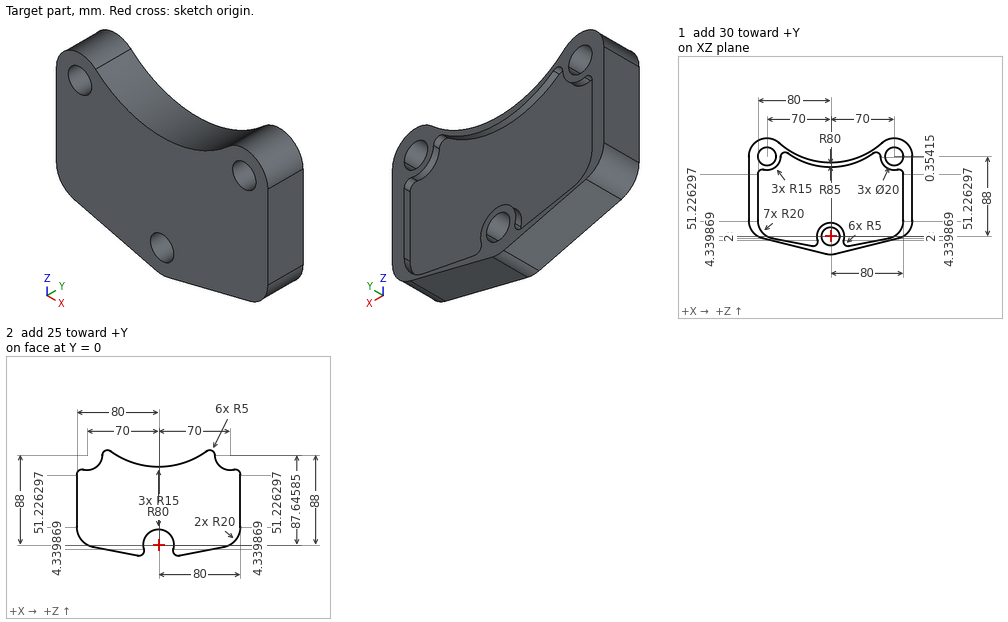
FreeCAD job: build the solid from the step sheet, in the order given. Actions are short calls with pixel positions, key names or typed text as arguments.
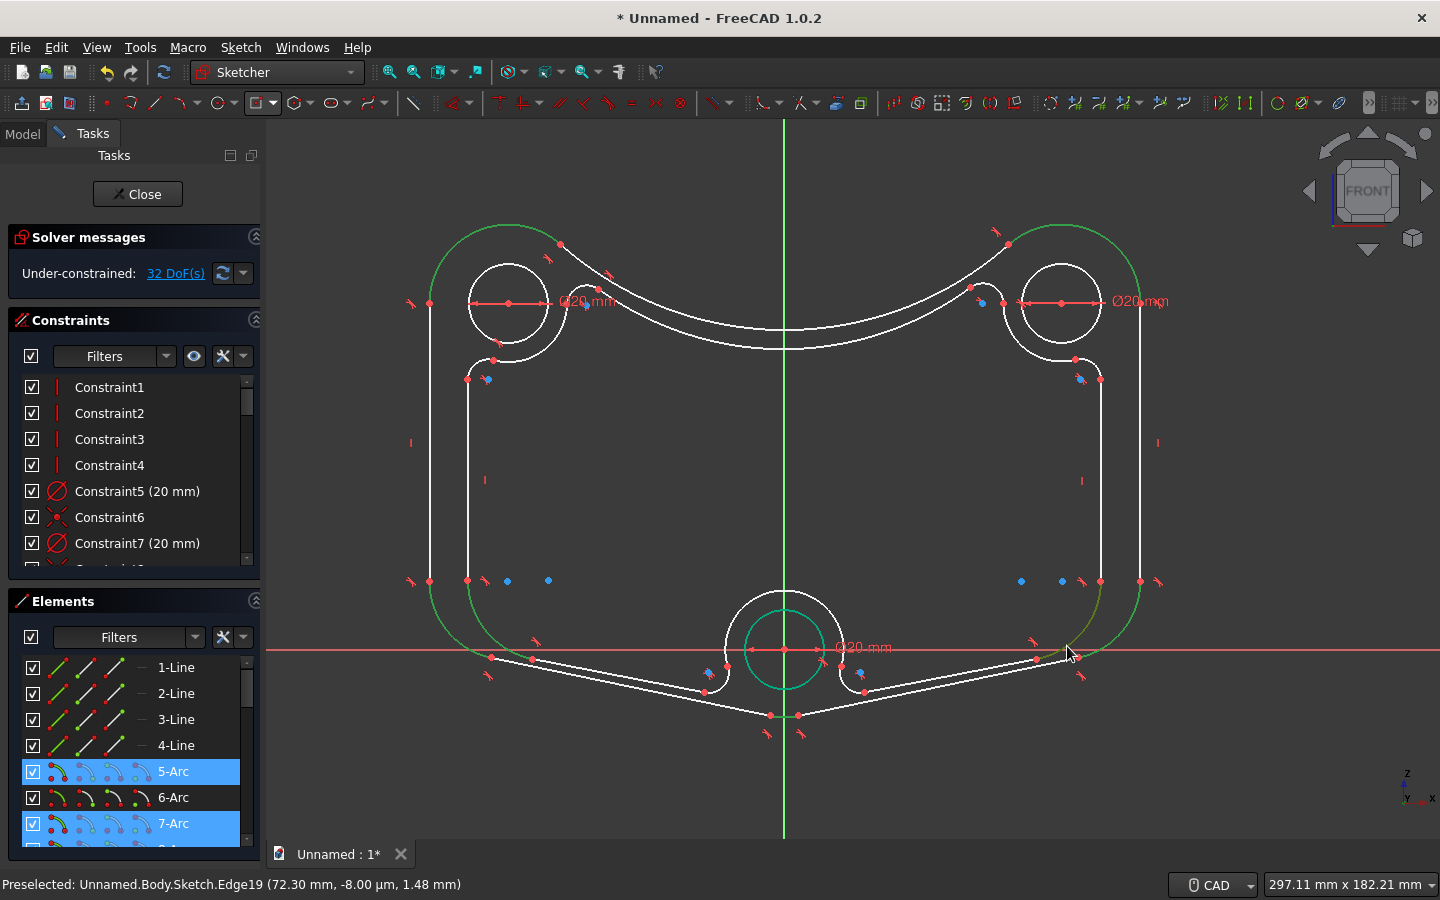
click(632, 104)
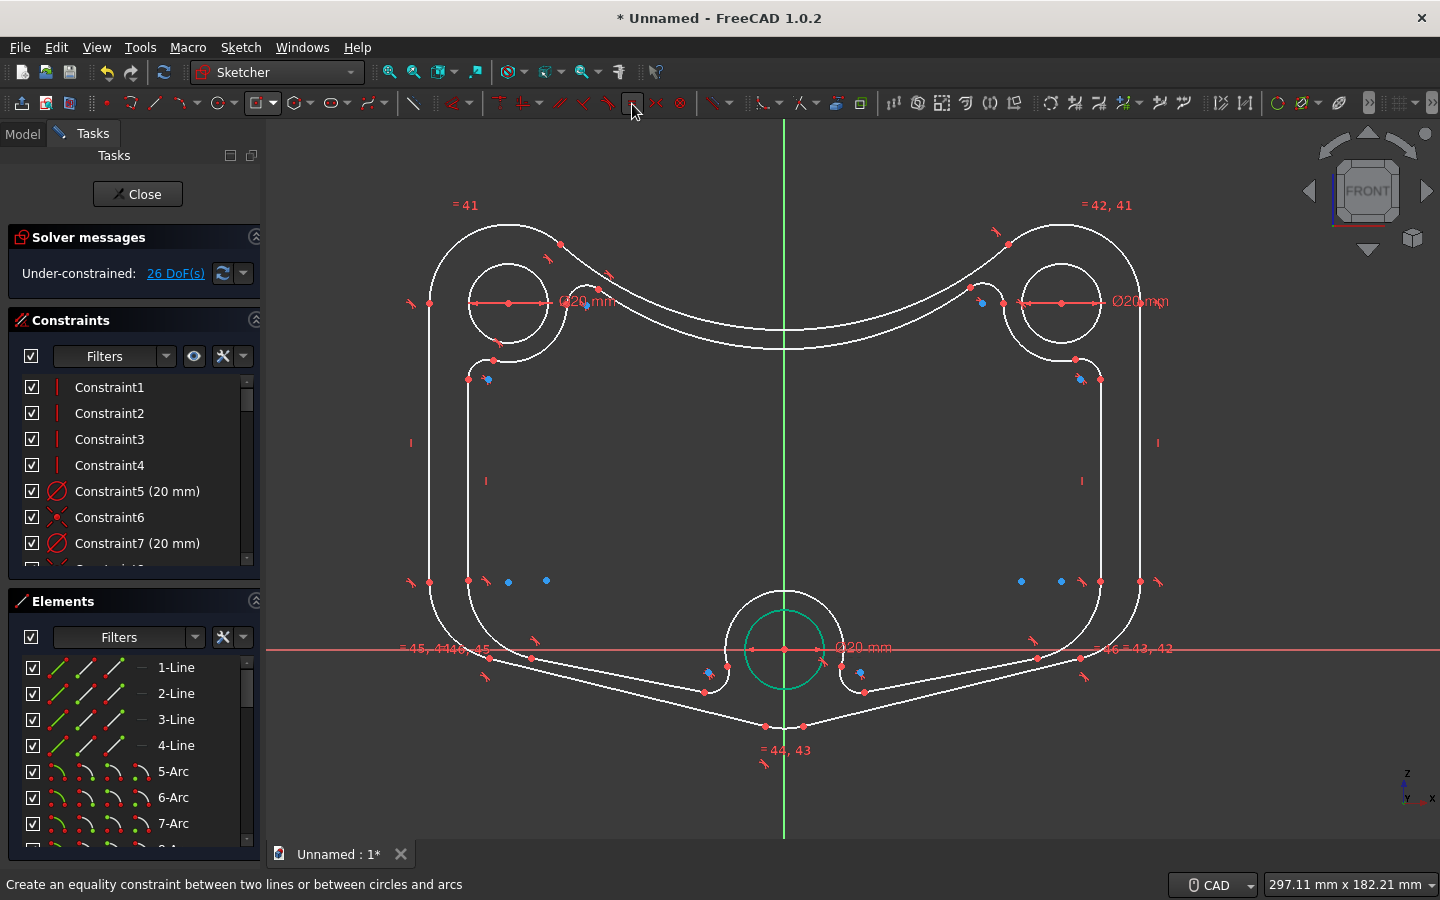
click(717, 691)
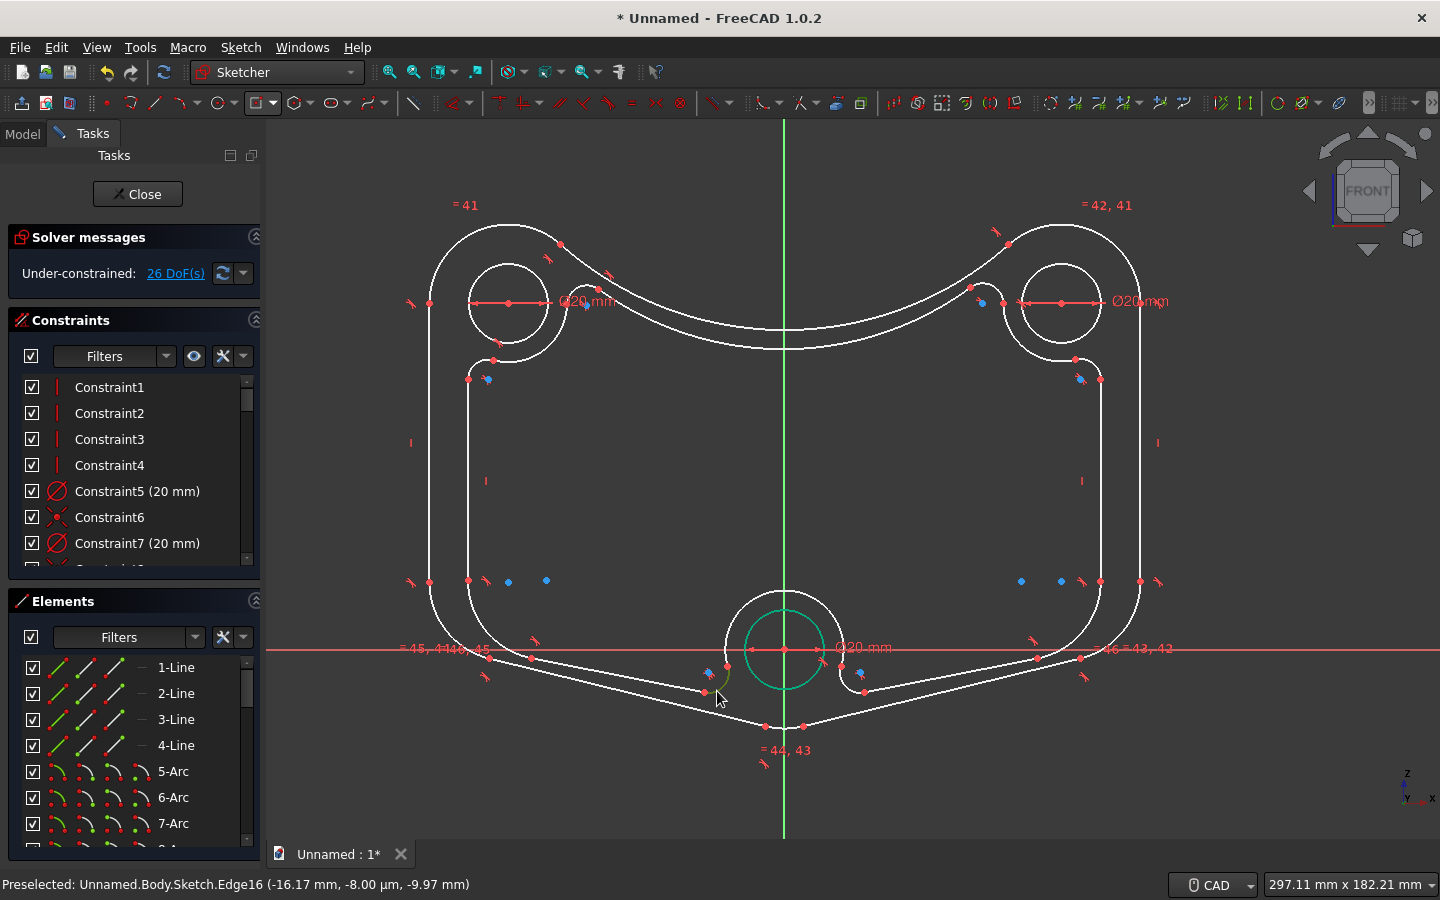
click(841, 679)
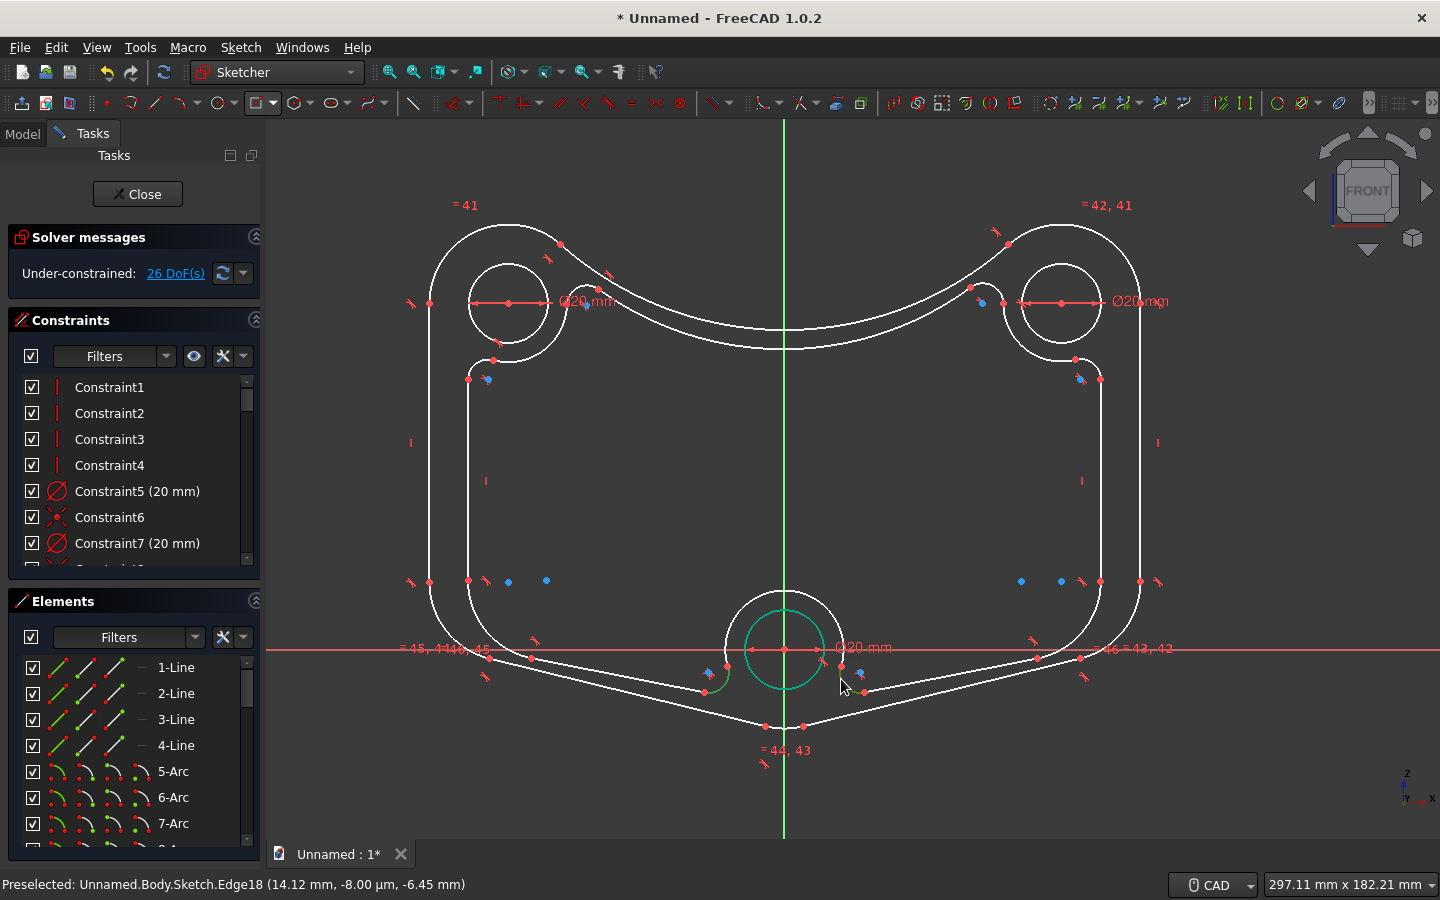
scroll(1098, 369, up, 2)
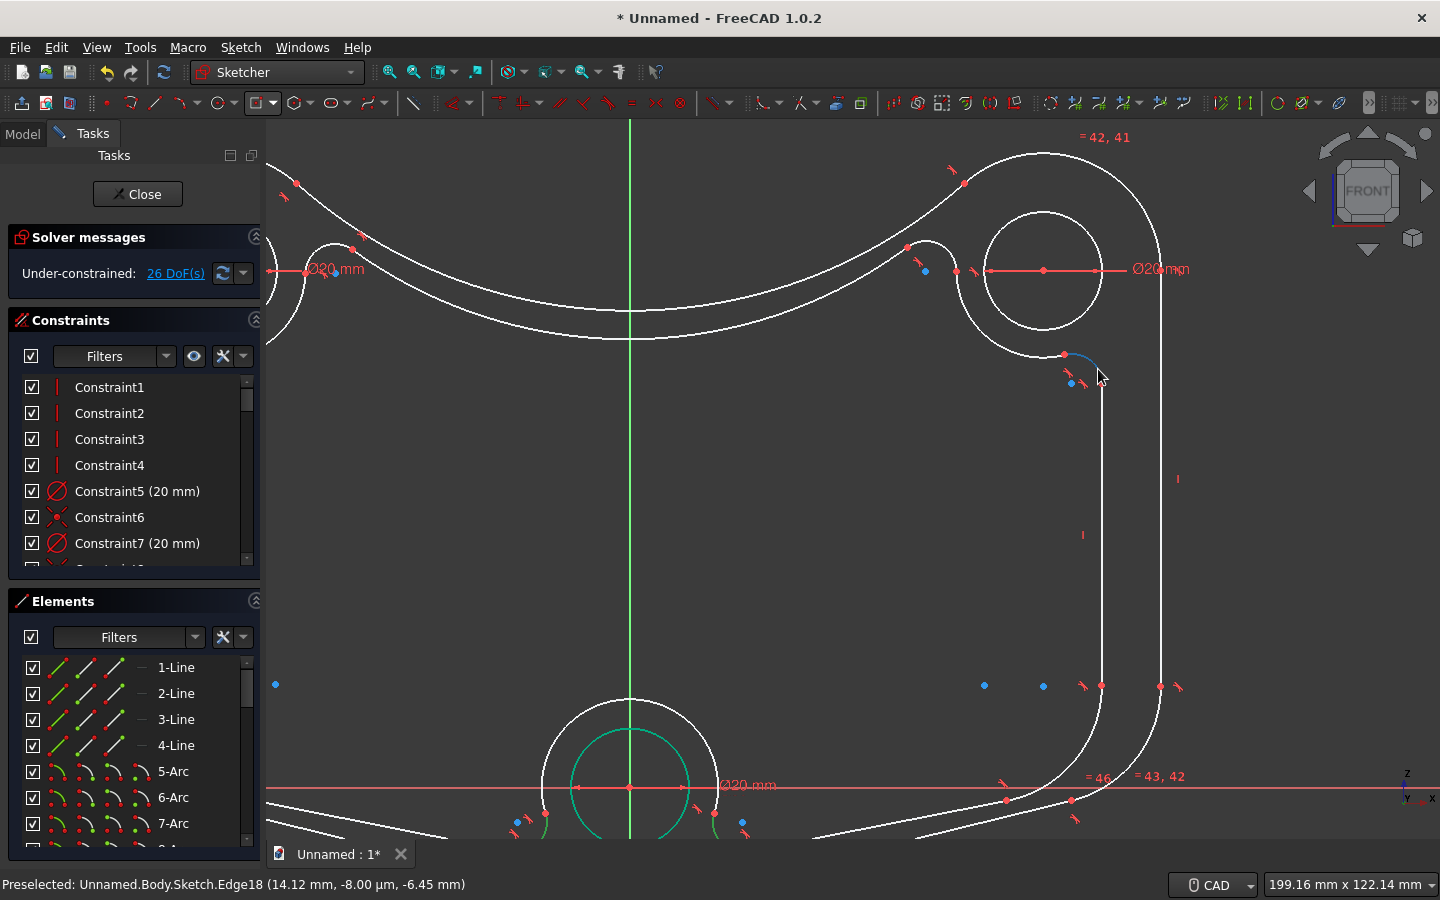
click(1098, 368)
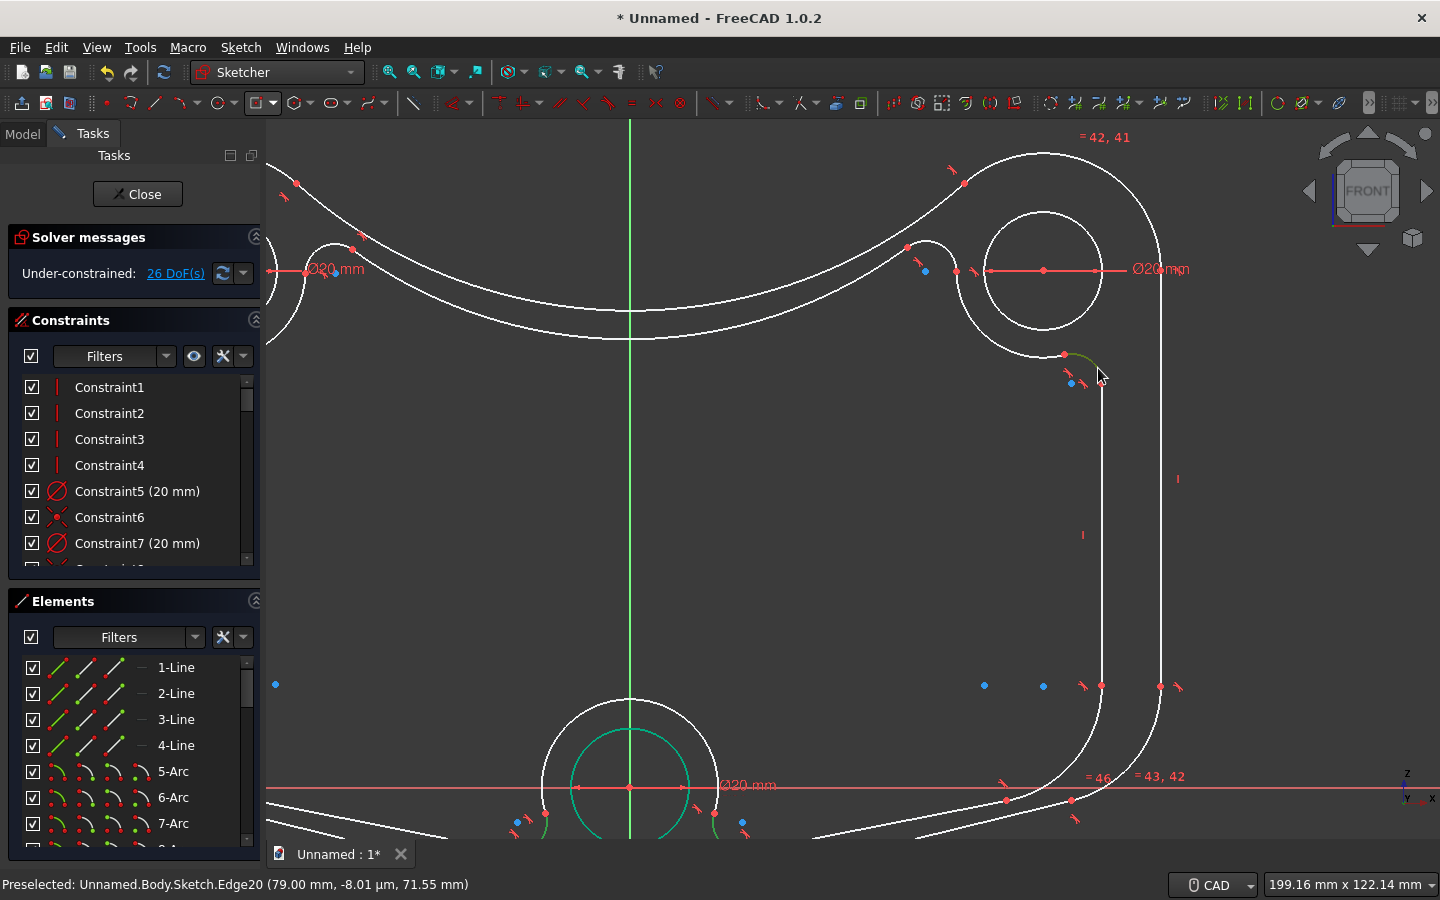
click(950, 253)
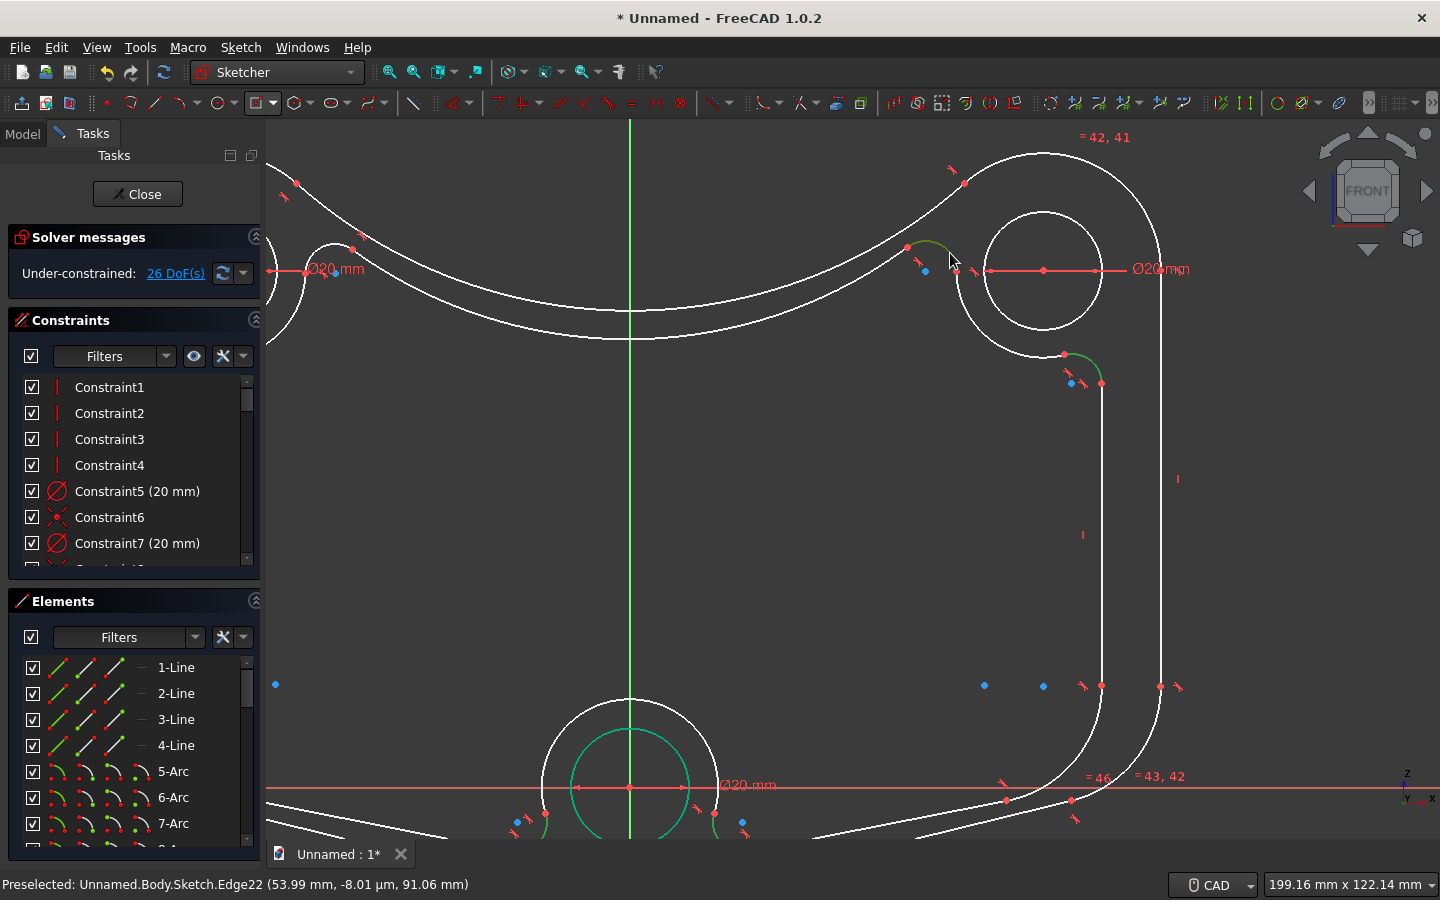
click(334, 244)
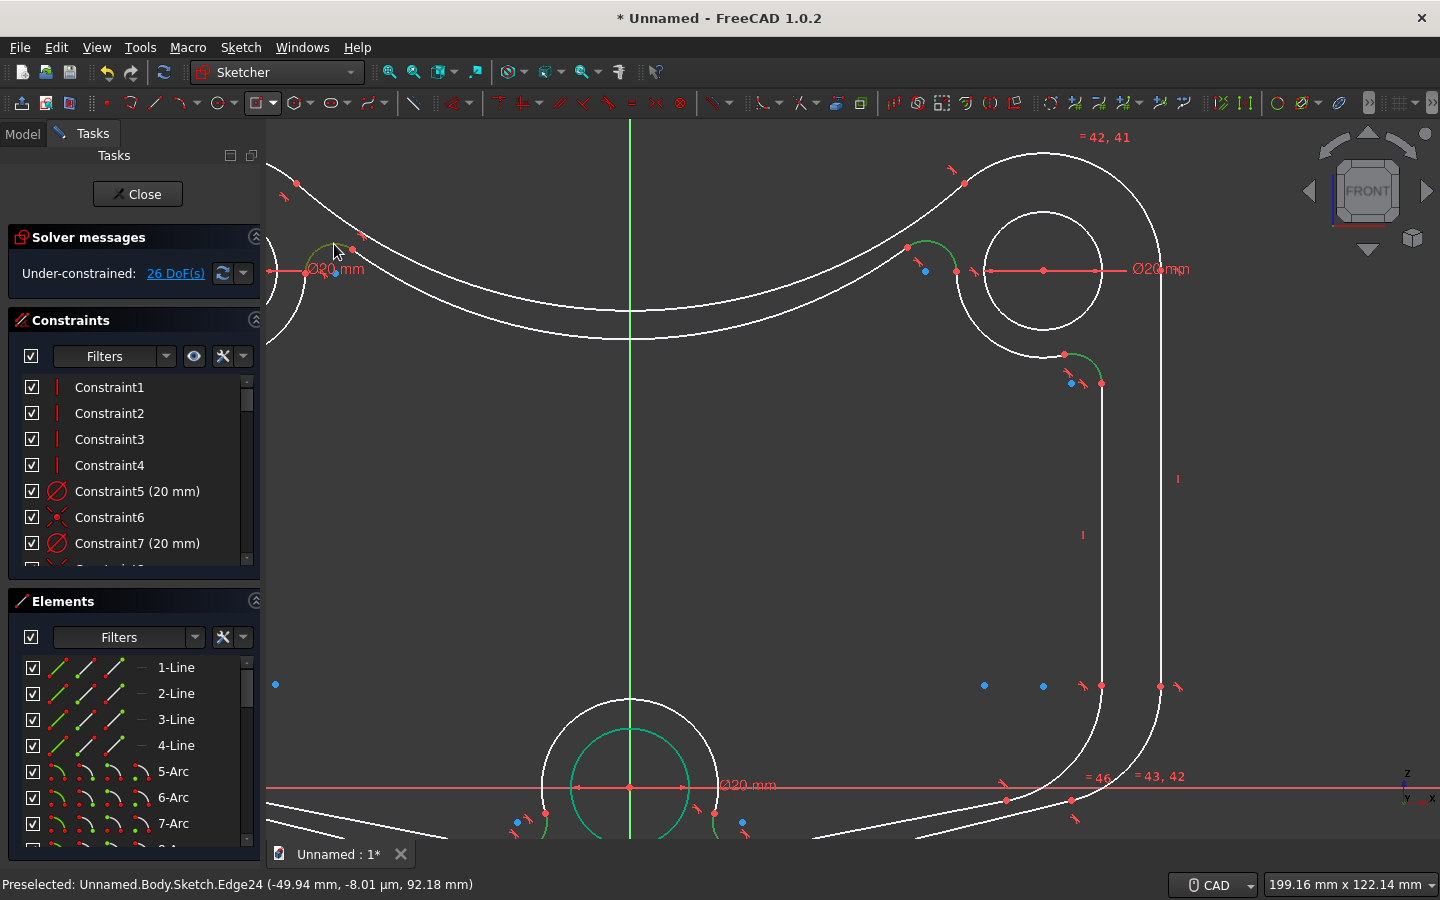
scroll(1099, 369, down, 2)